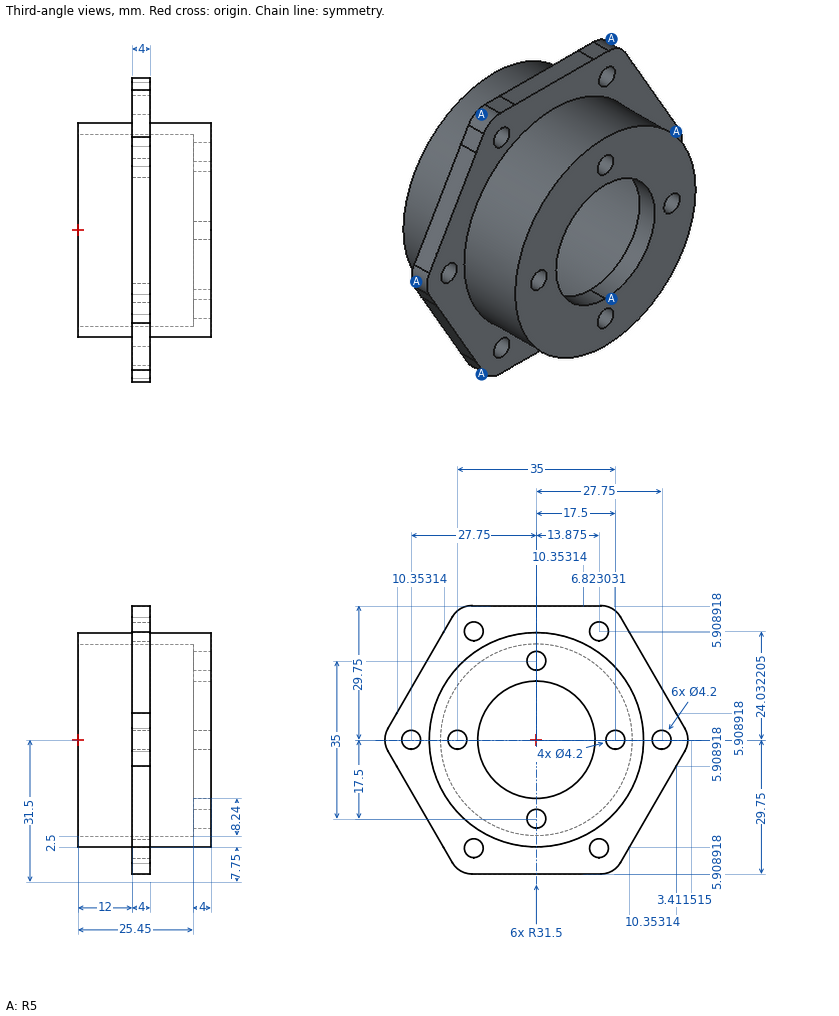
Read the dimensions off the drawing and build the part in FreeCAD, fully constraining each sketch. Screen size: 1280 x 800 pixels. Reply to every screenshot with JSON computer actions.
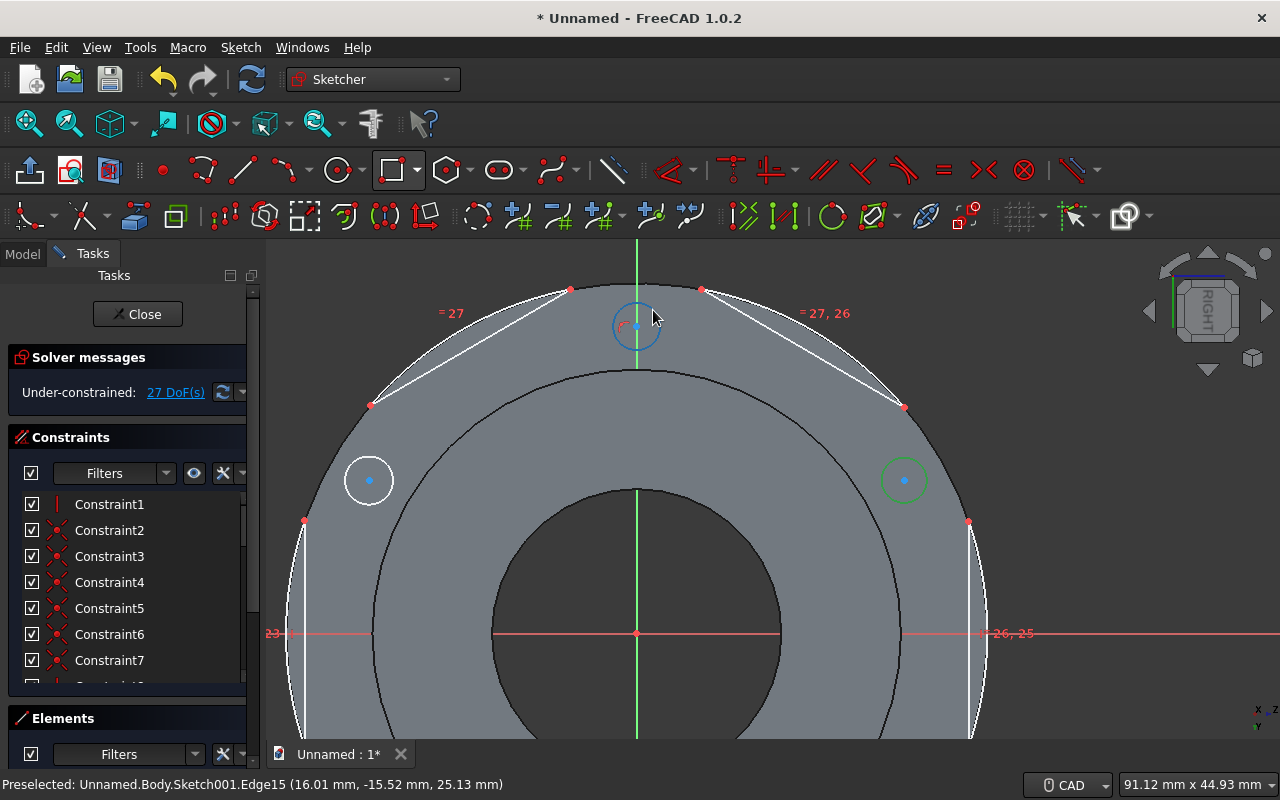
{"action": "left_click", "coordinate": [653, 310]}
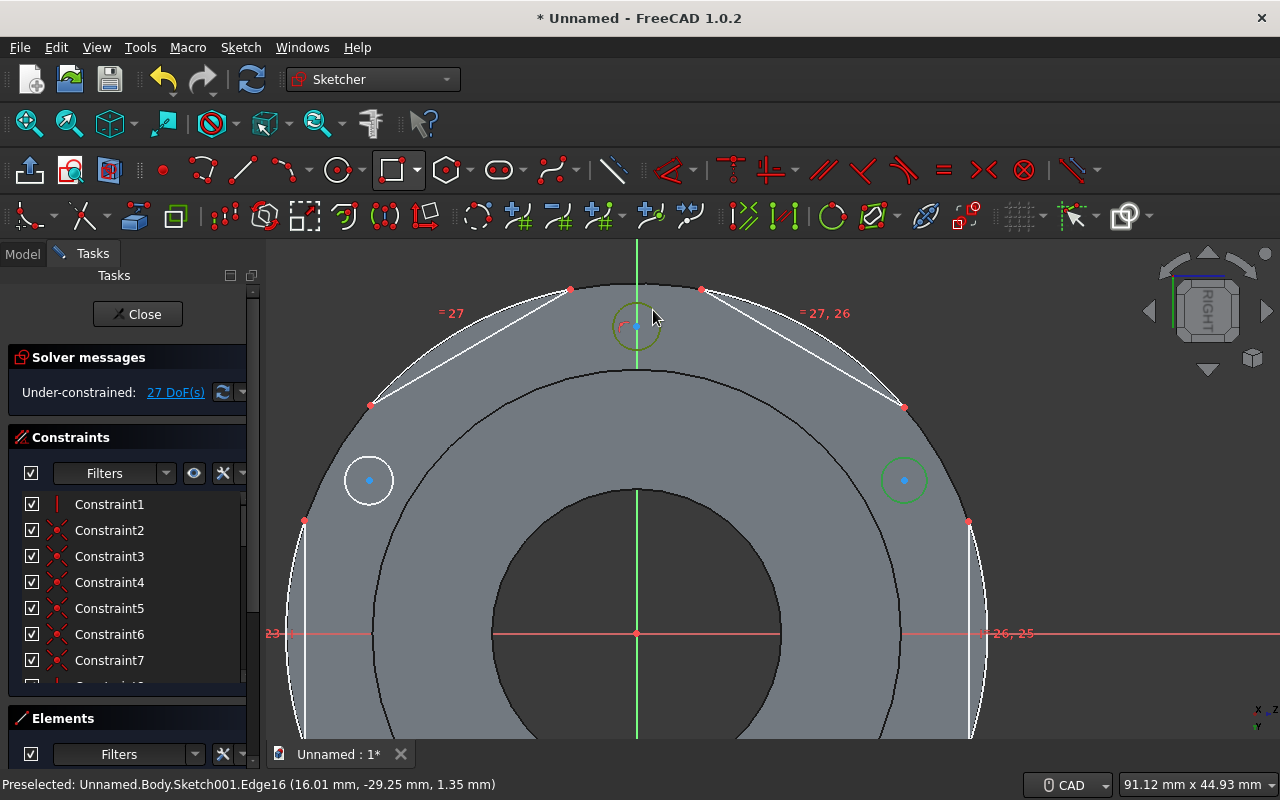
{"action": "left_click", "coordinate": [386, 463]}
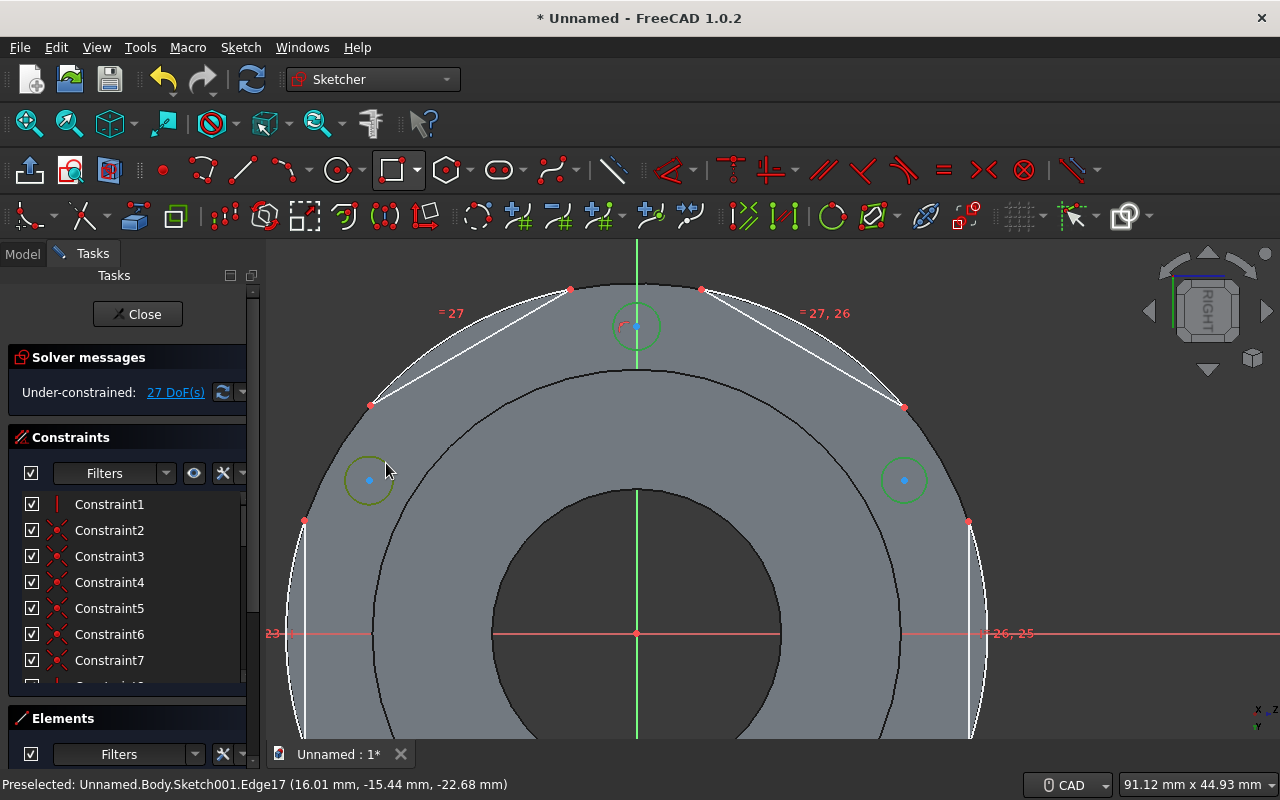
{"action": "scroll", "coordinate": [760, 371], "scroll_direction": "down", "scroll_amount": 4}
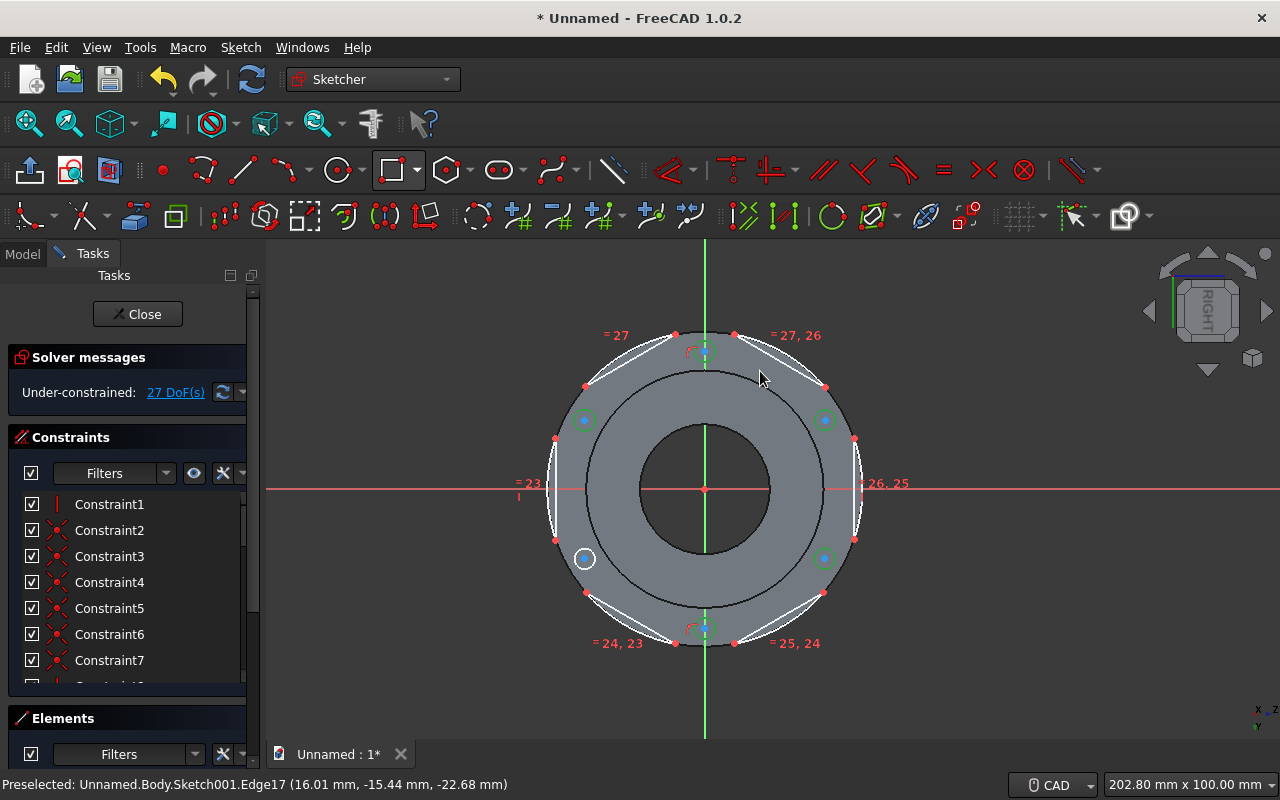
{"action": "scroll", "coordinate": [592, 552], "scroll_direction": "up", "scroll_amount": 2}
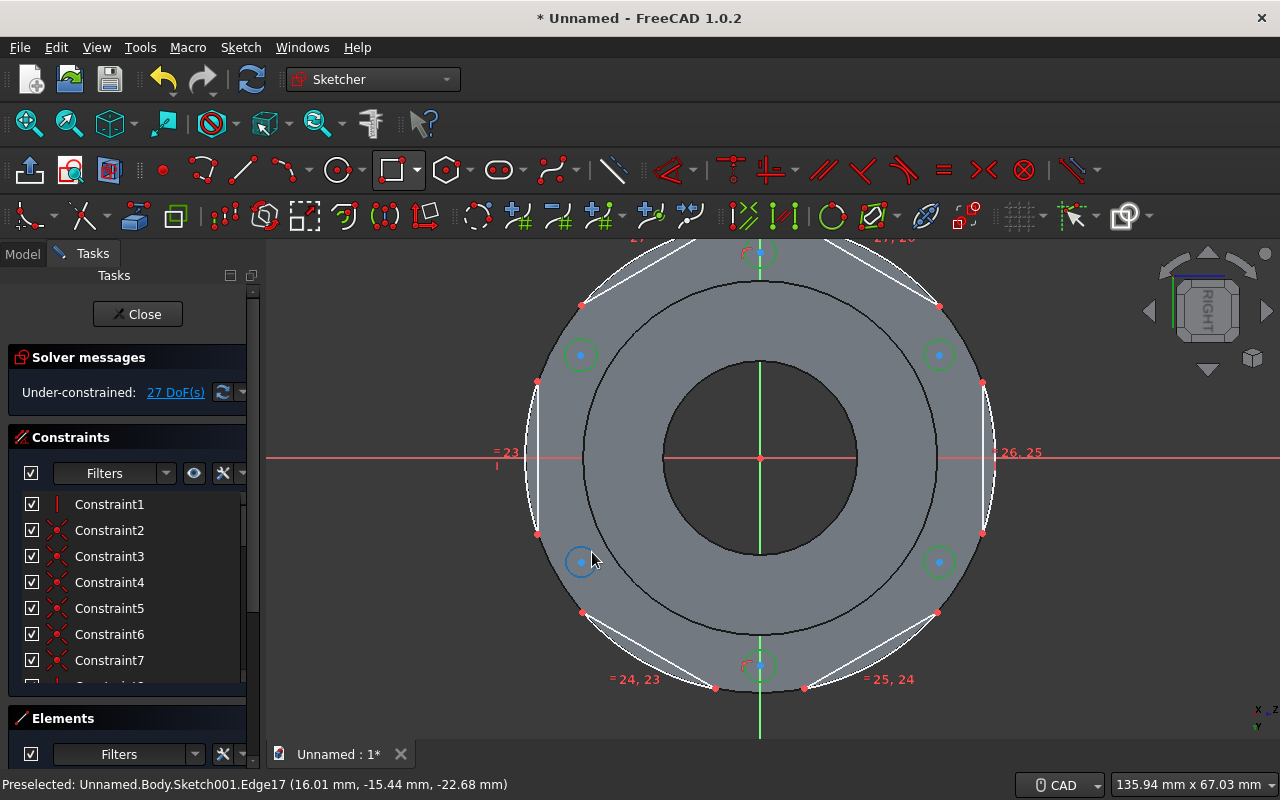
{"action": "left_click", "coordinate": [592, 551]}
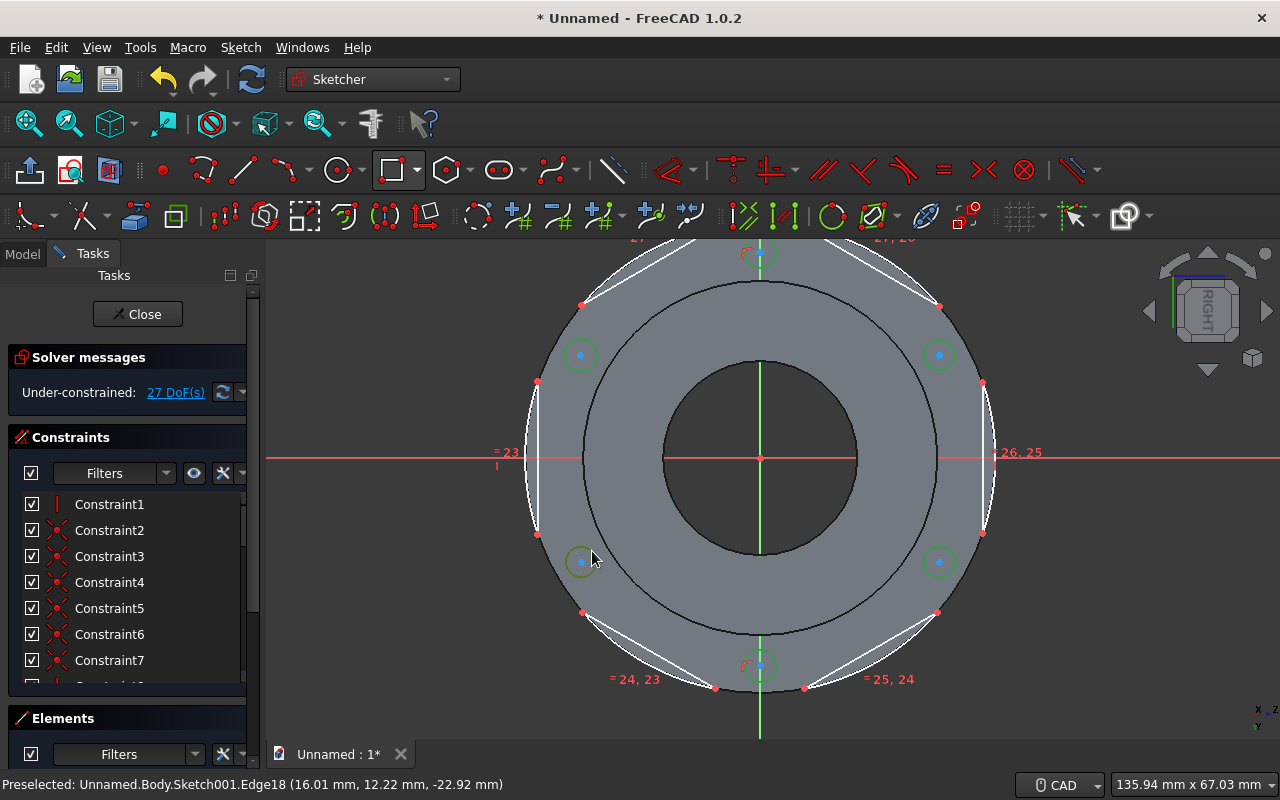
{"action": "key", "text": "e"}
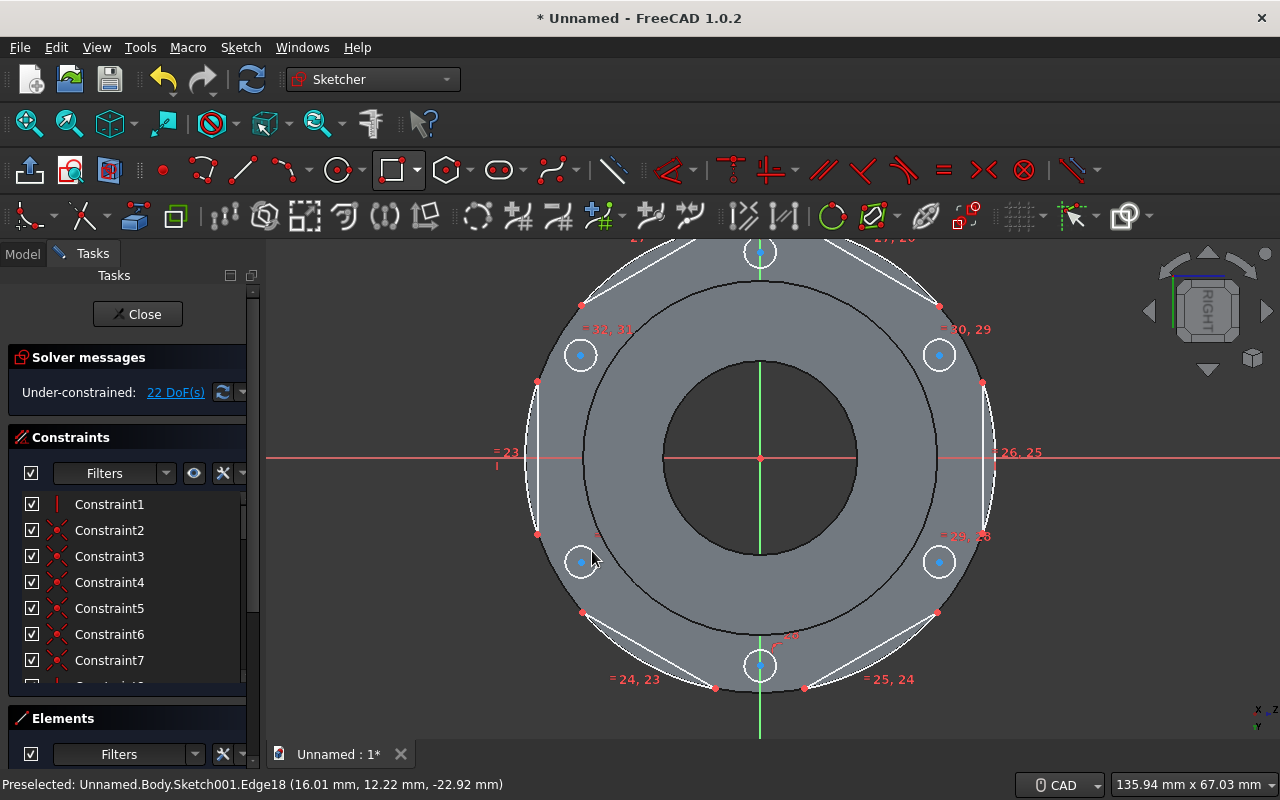
{"action": "left_click", "coordinate": [939, 562]}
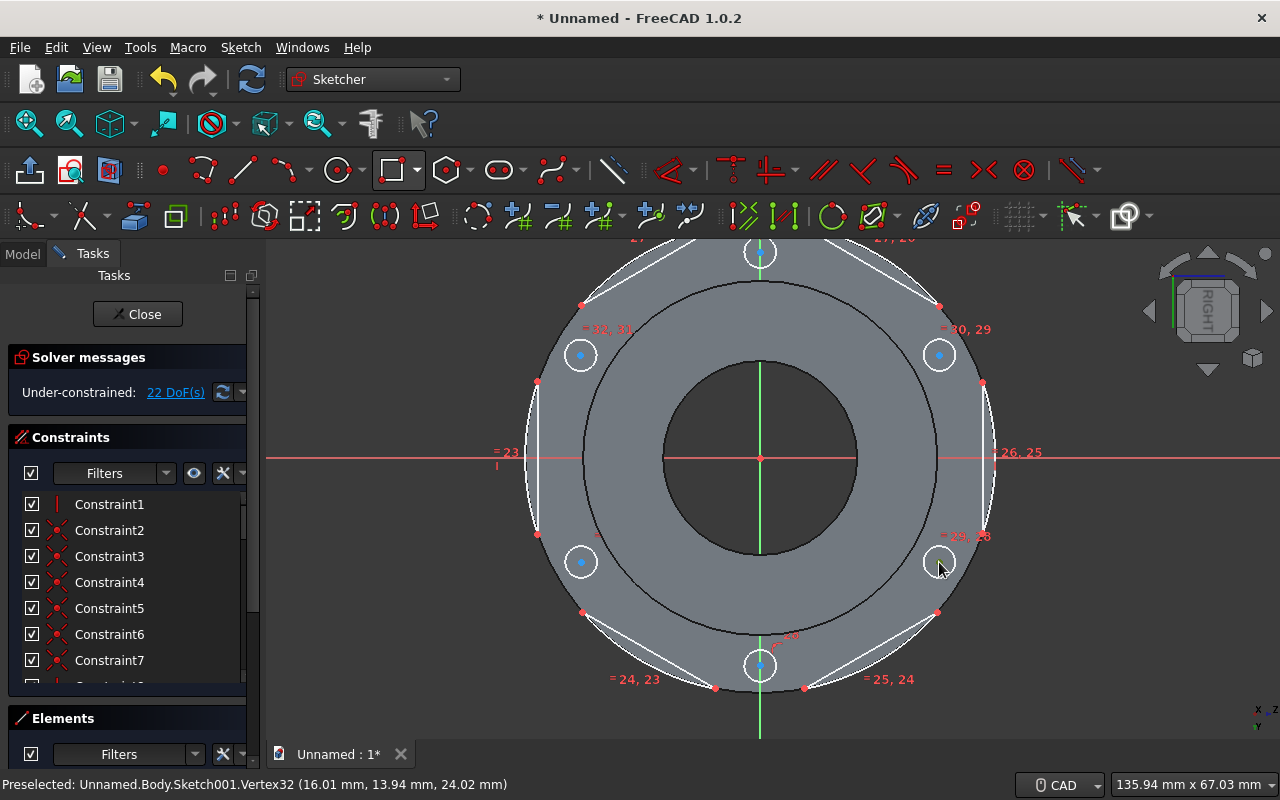
{"action": "left_click", "coordinate": [940, 355]}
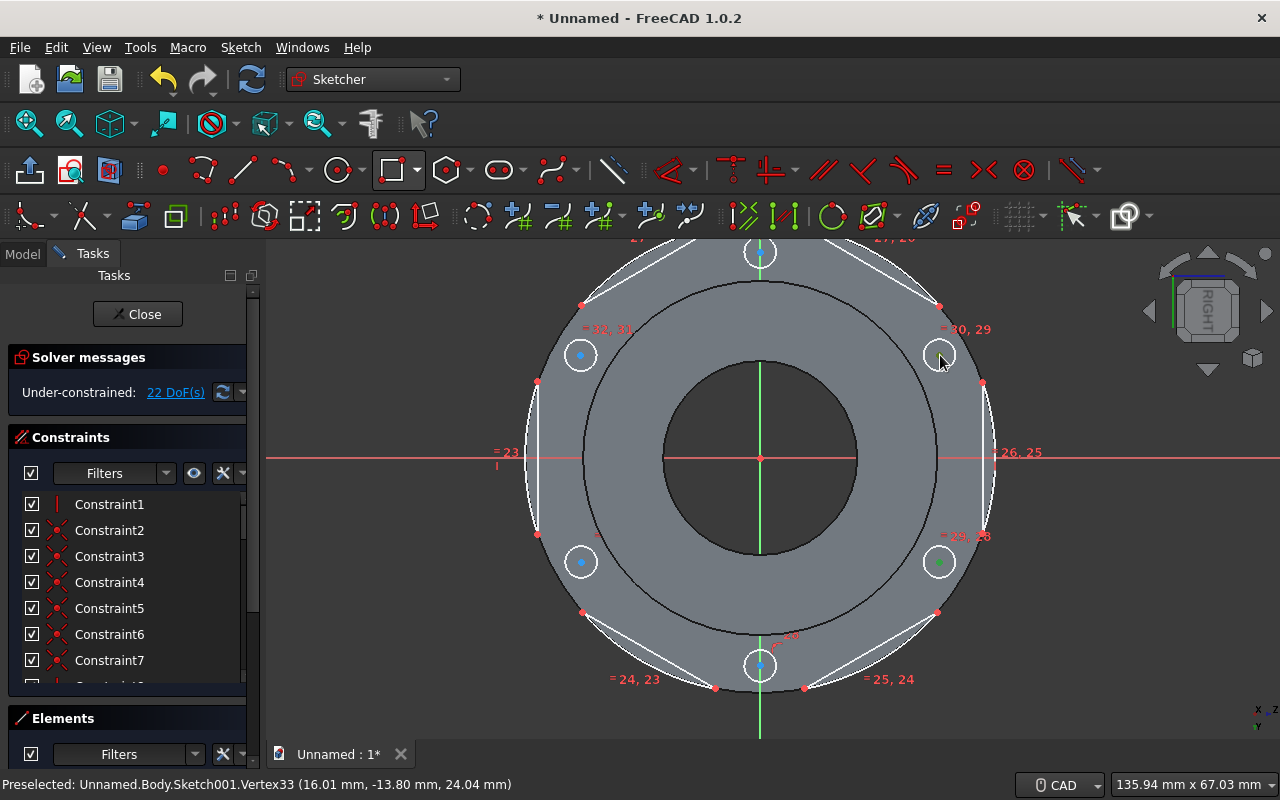
{"action": "left_click", "coordinate": [353, 458]}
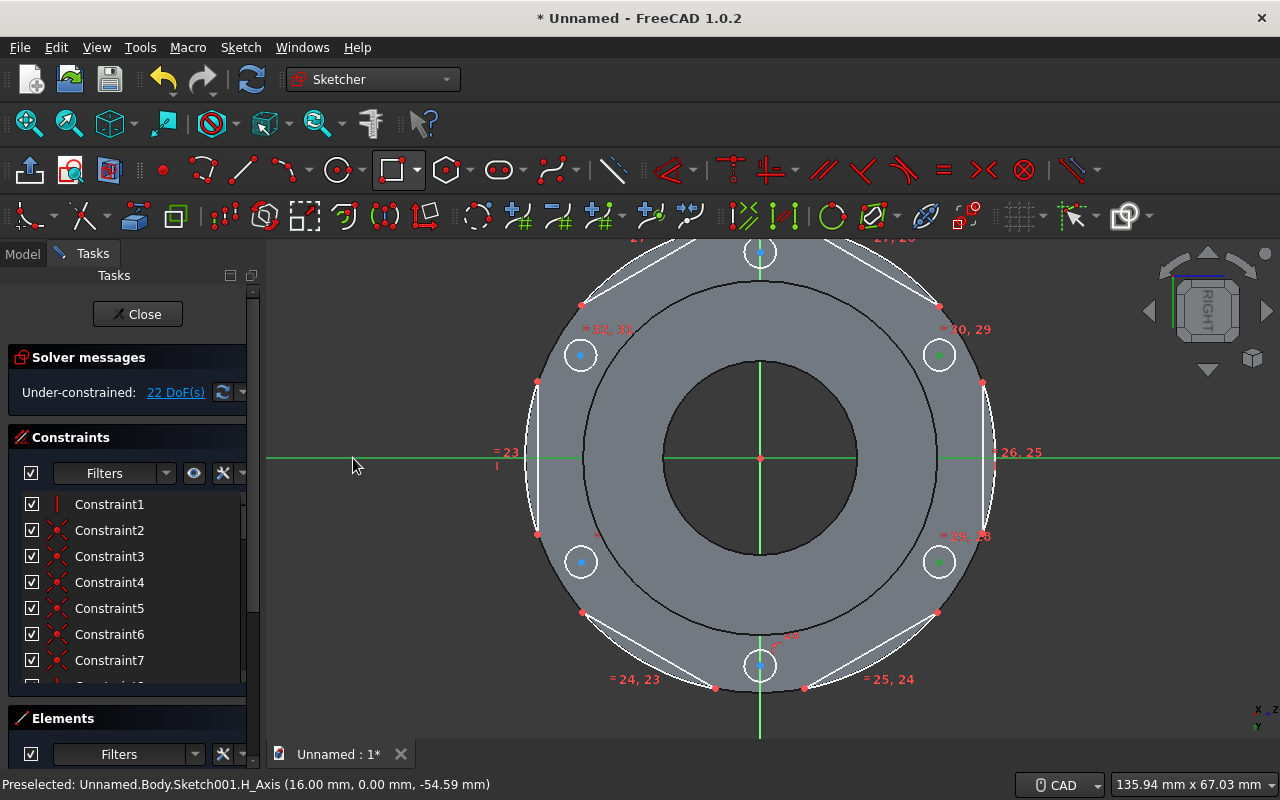
{"action": "key", "text": "s"}